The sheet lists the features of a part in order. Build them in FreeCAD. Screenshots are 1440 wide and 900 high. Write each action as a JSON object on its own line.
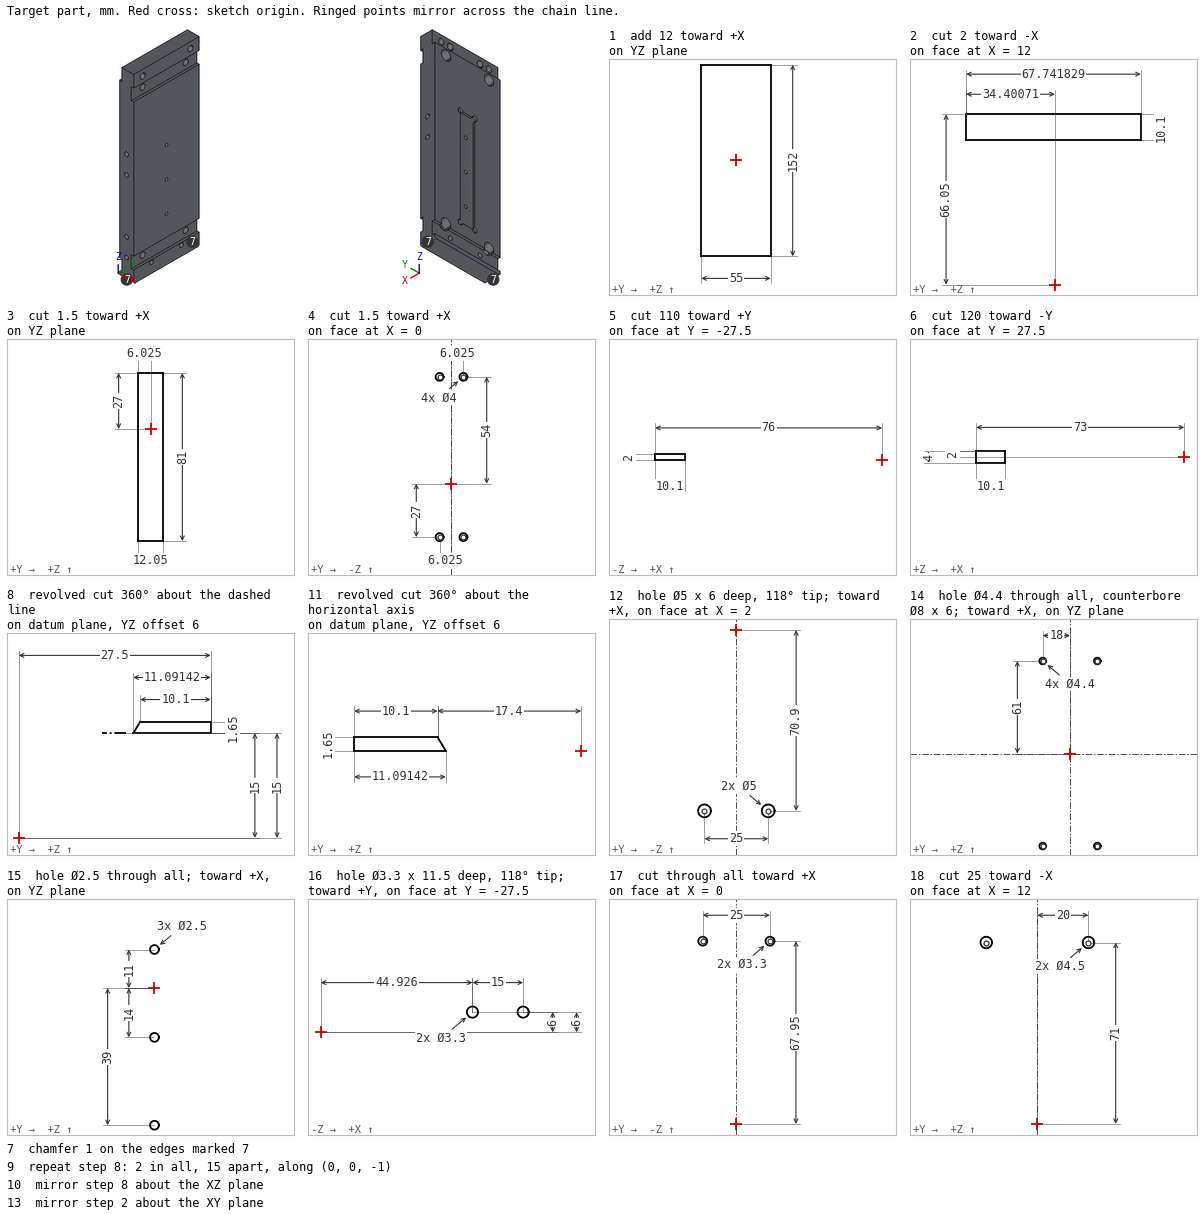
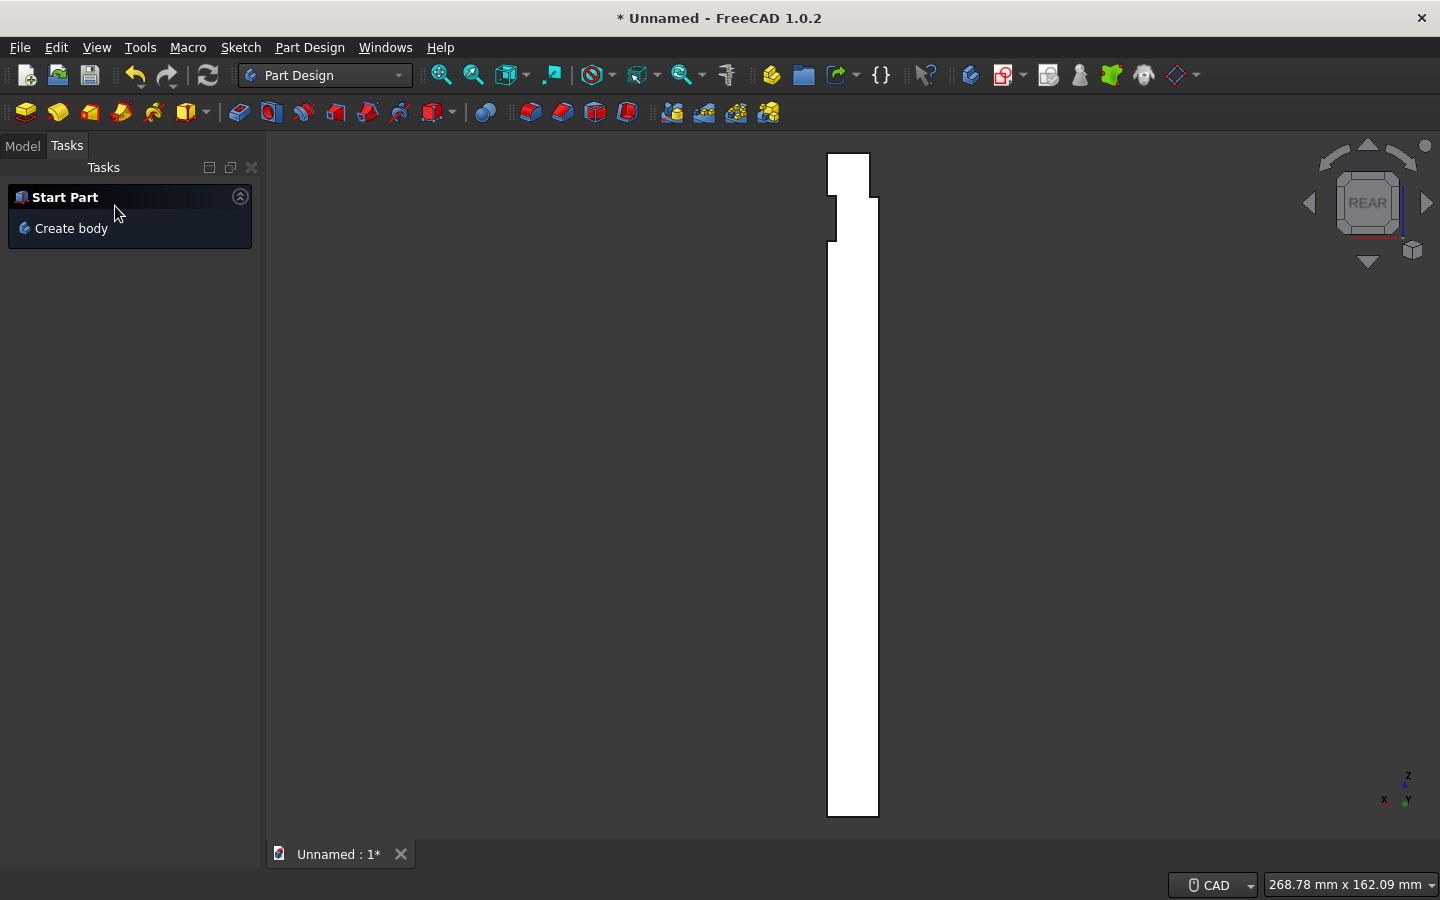
{"action": "left_click", "coordinate": [853, 769]}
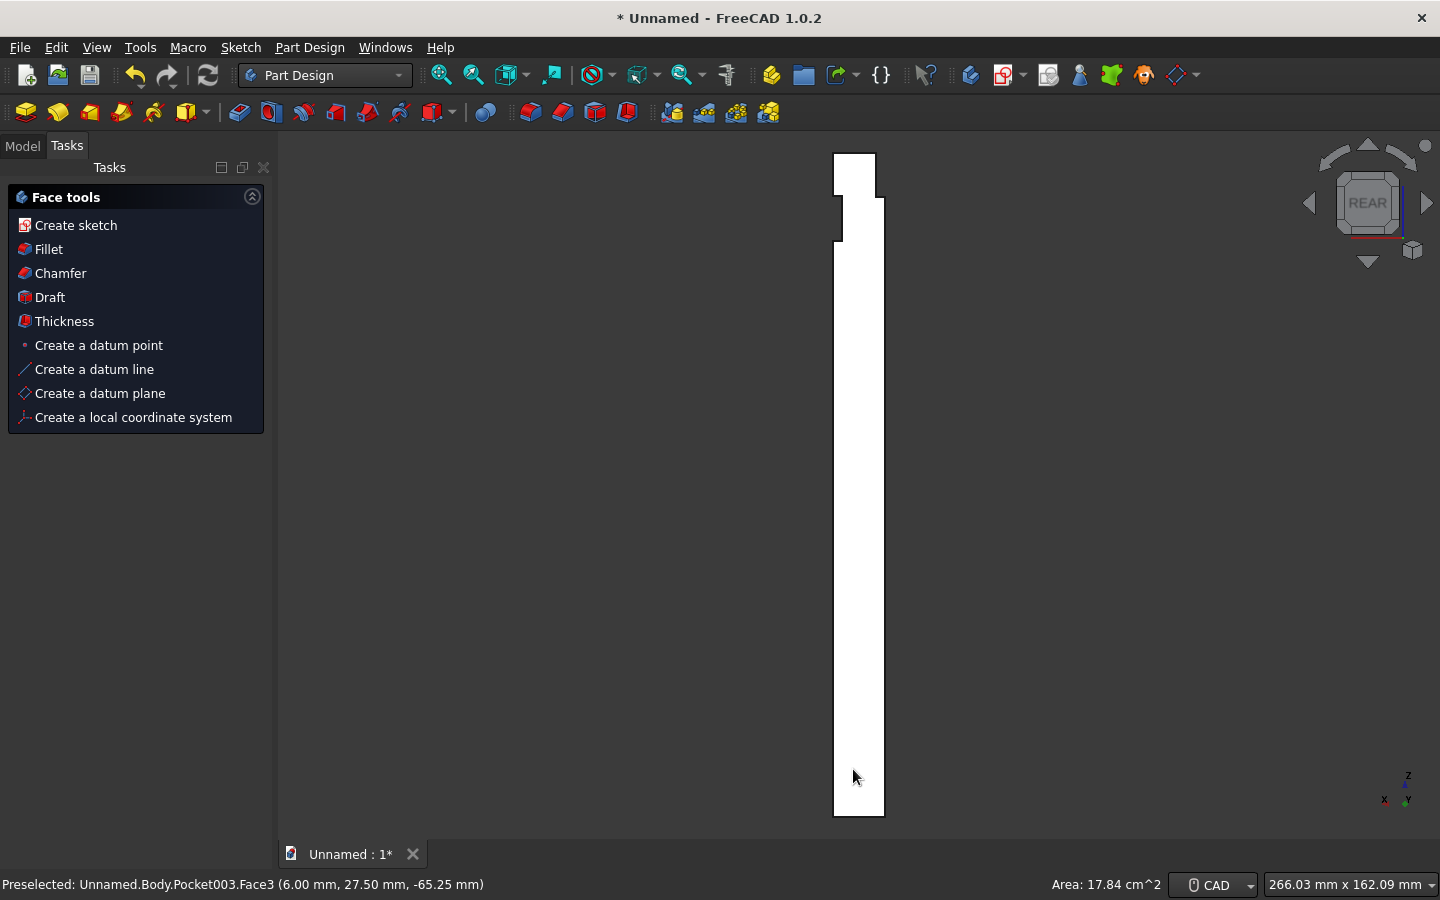
{"action": "left_click", "coordinate": [1004, 76]}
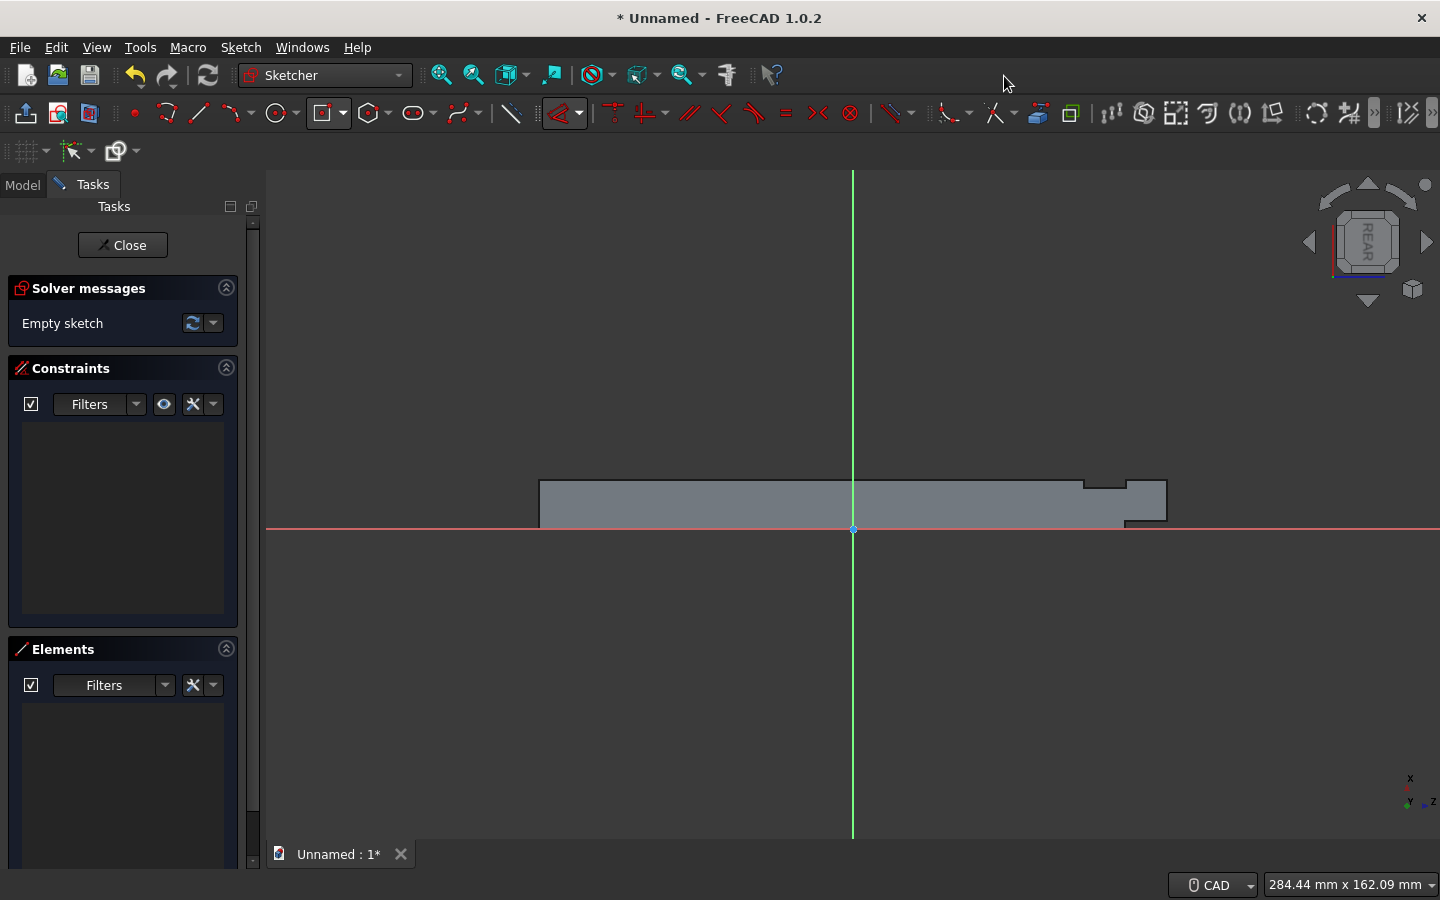
{"action": "scroll", "coordinate": [559, 531], "scroll_direction": "up", "scroll_amount": 14}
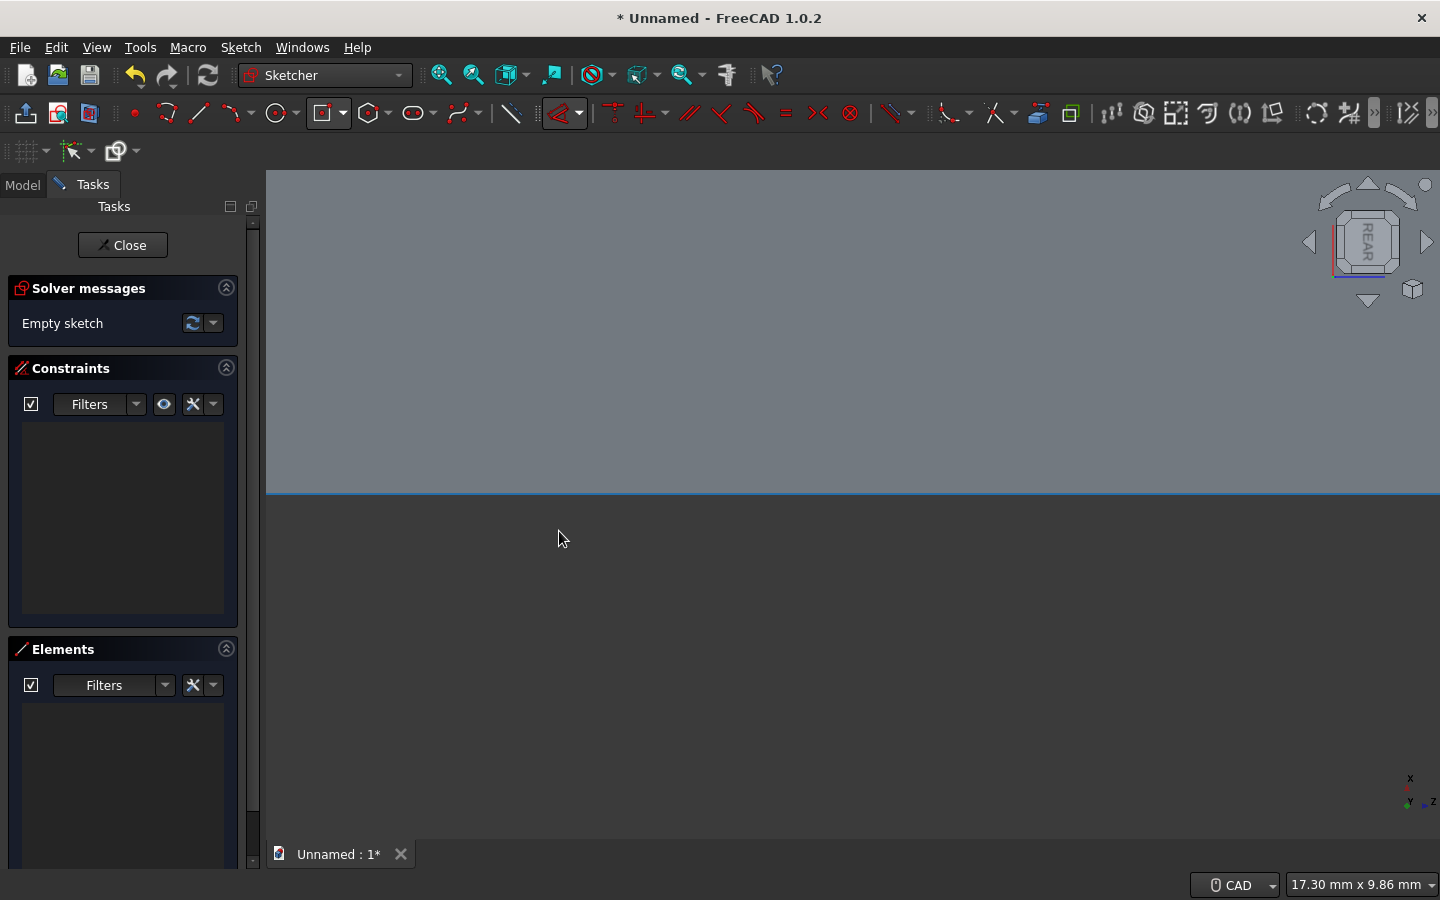
{"action": "key", "text": "g r"}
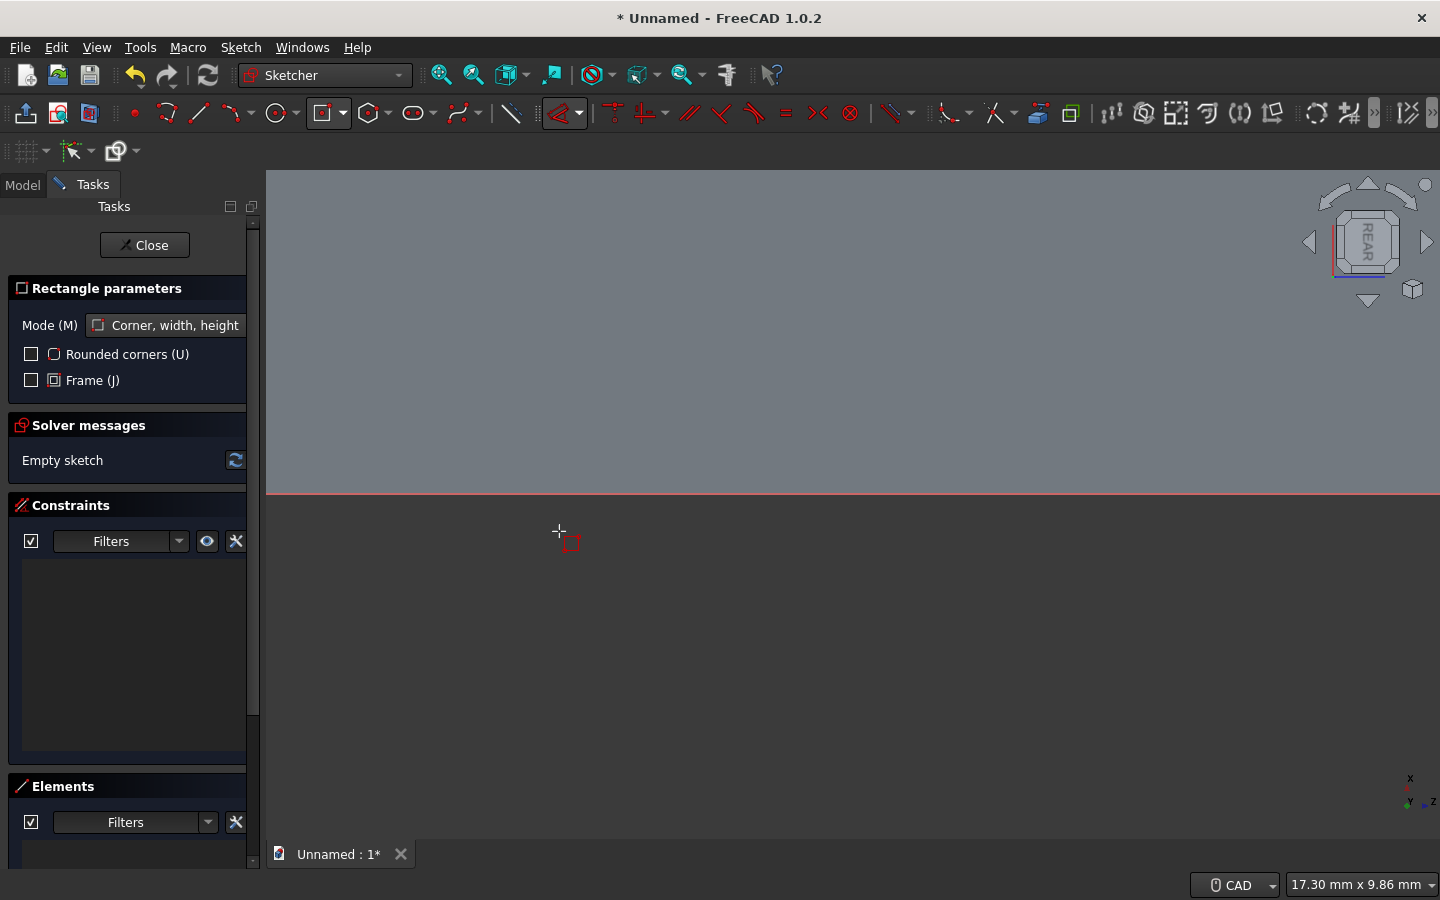
{"action": "left_click", "coordinate": [435, 358]}
{"action": "mouse_move", "coordinate": [1121, 630]}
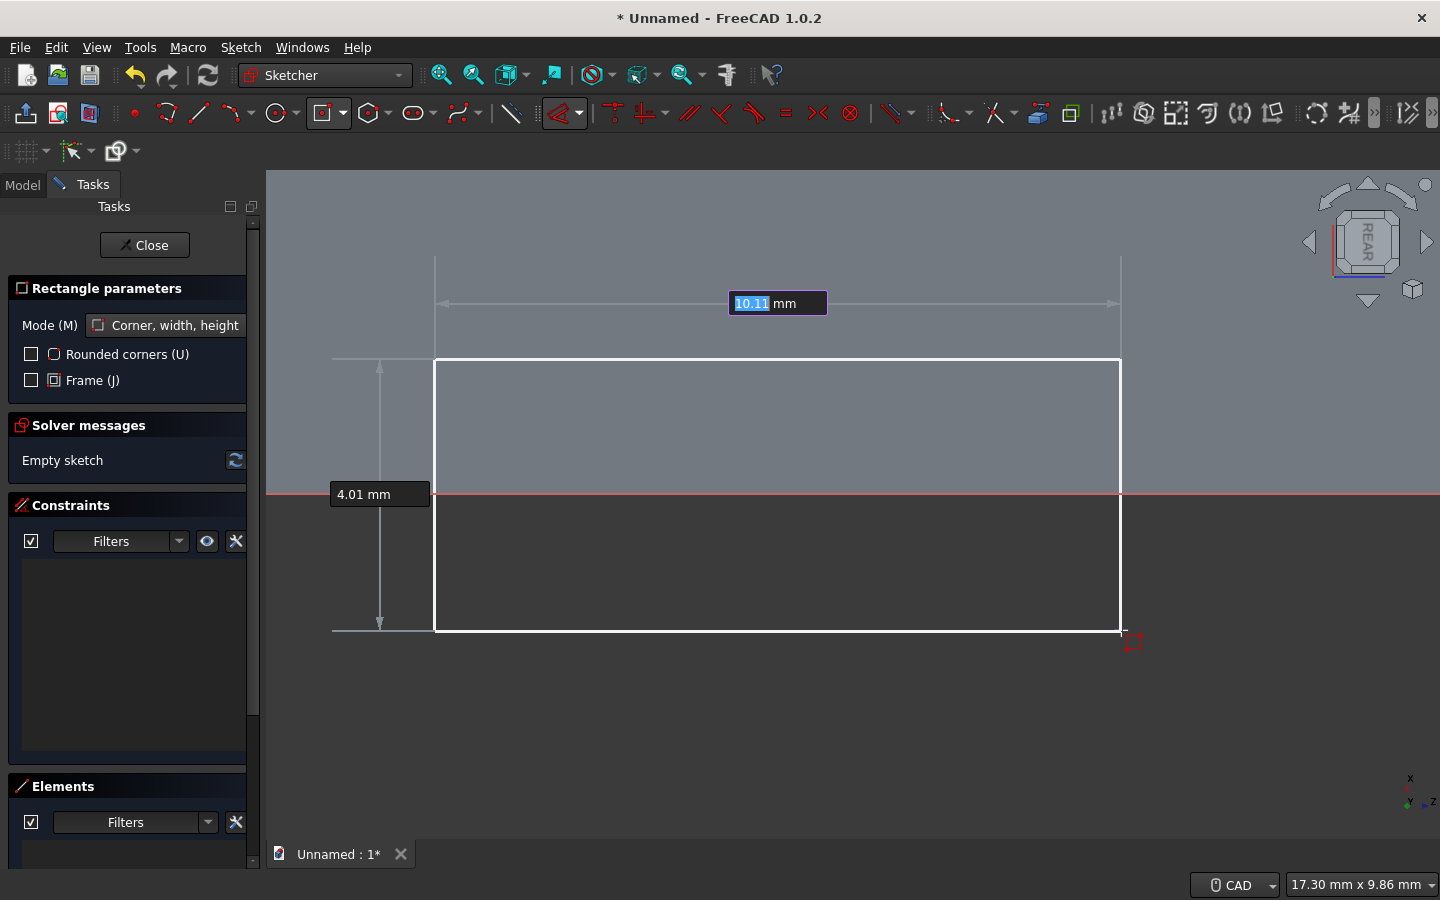
{"action": "type", "text": "10.1"}
{"action": "key", "text": "Tab"}
{"action": "type", "text": "4"}
{"action": "key", "text": "Return"}
{"action": "key", "text": "Escape"}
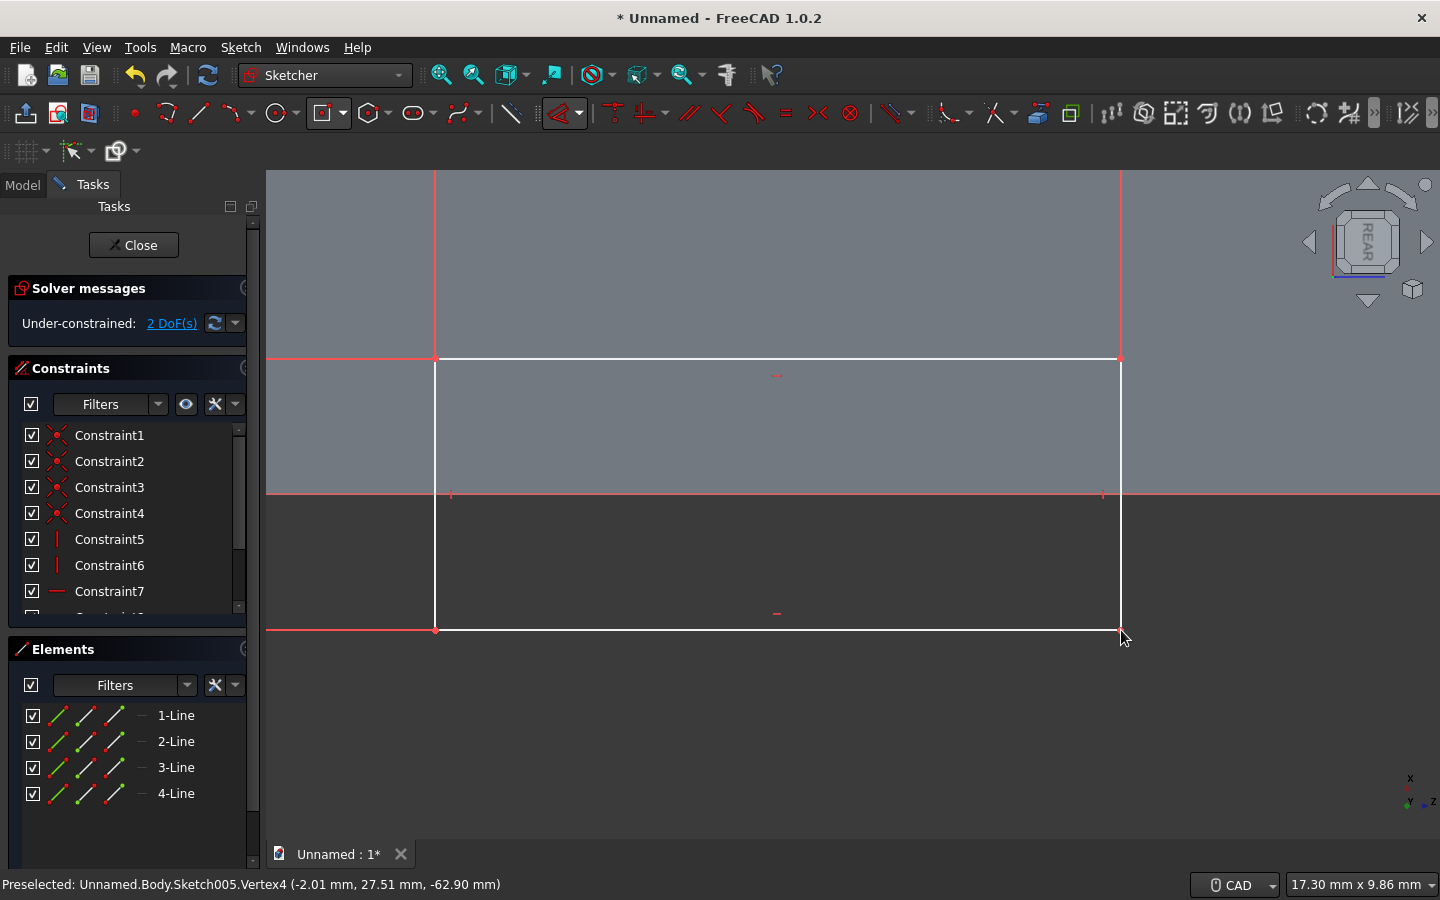
{"action": "left_click", "coordinate": [435, 359]}